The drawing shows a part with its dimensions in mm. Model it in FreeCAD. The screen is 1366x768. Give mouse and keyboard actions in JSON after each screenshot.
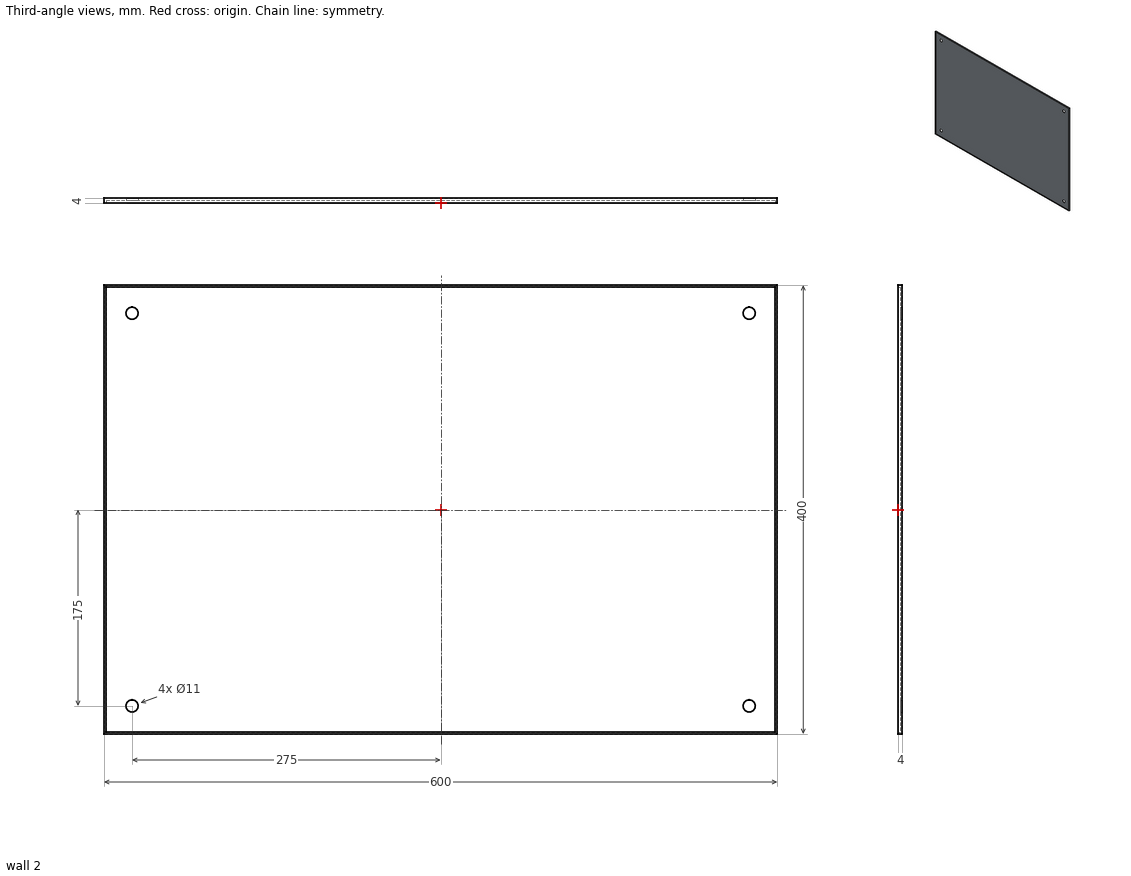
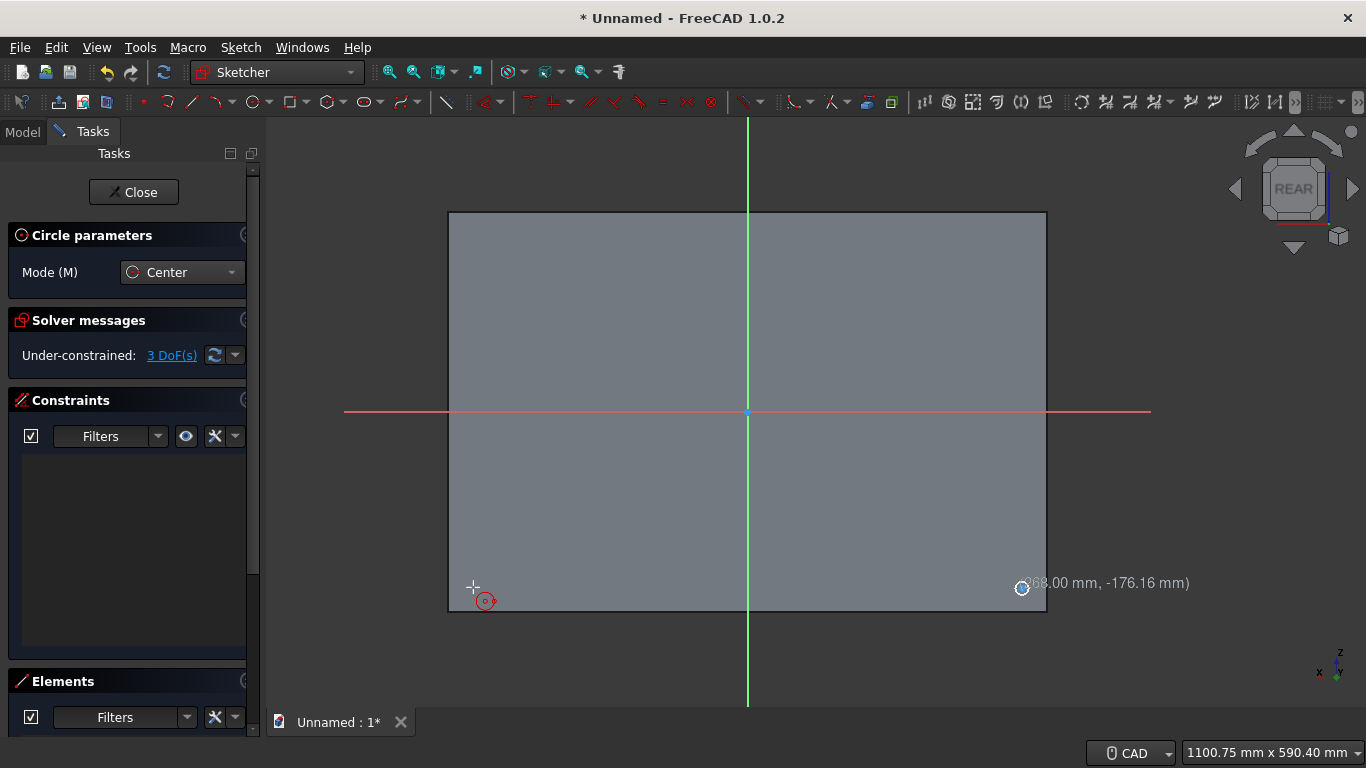
{"action": "left_click", "coordinate": [473, 587]}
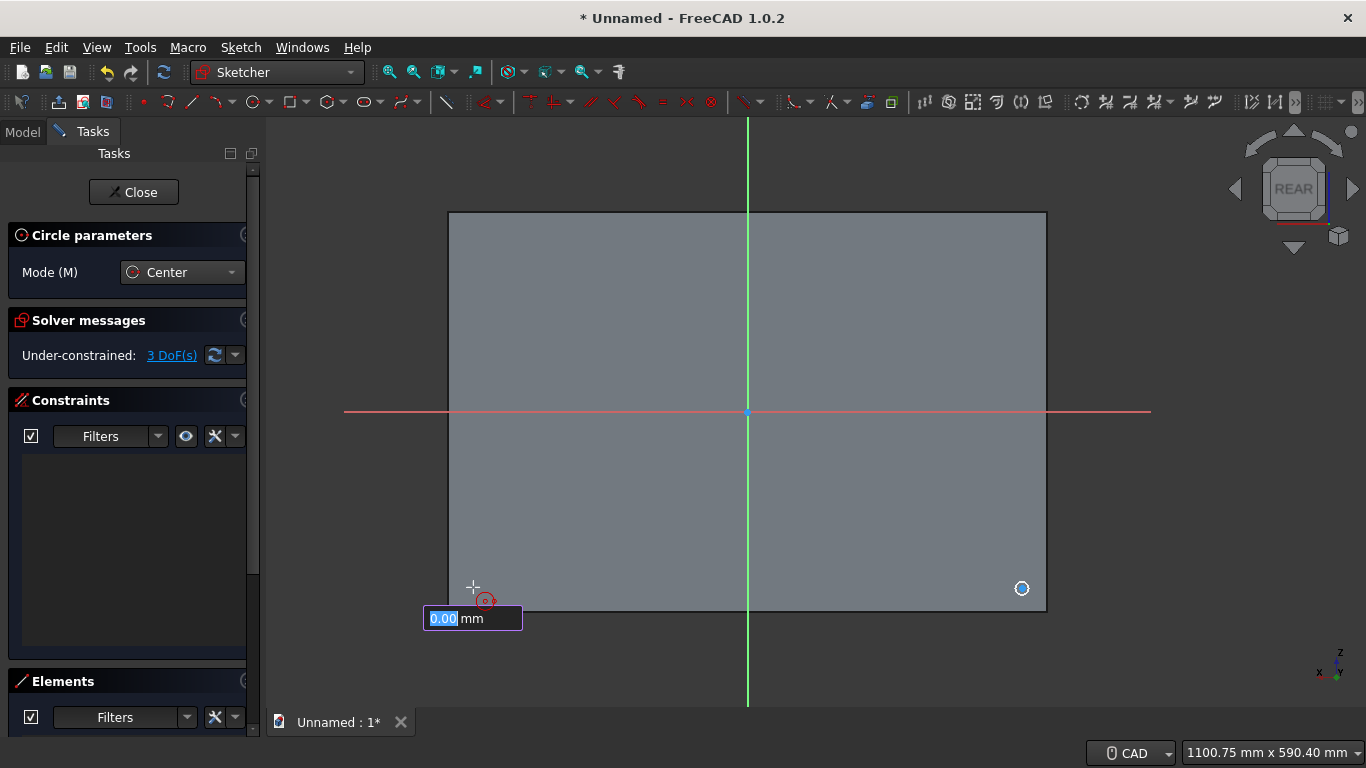
{"action": "scroll", "coordinate": [477, 583], "scroll_direction": "up", "scroll_amount": 6}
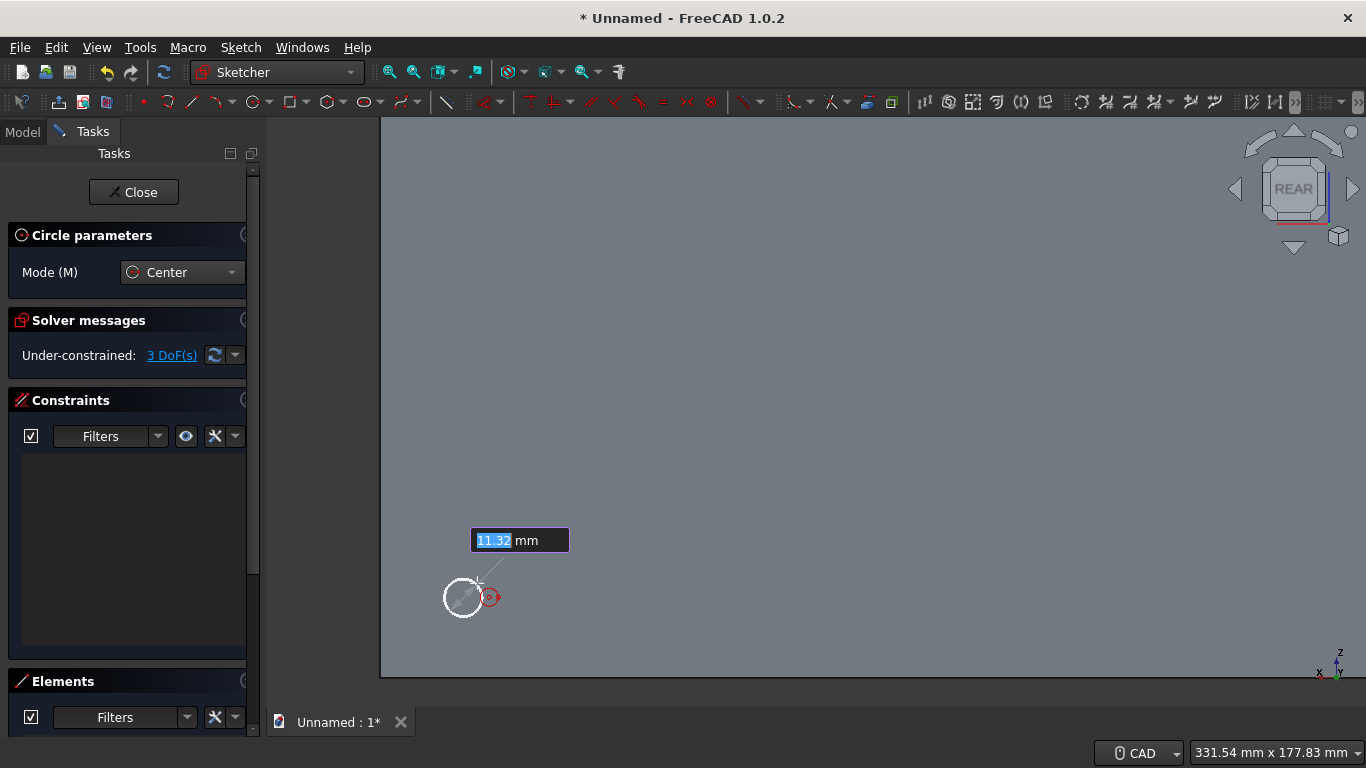
{"action": "left_click", "coordinate": [476, 582]}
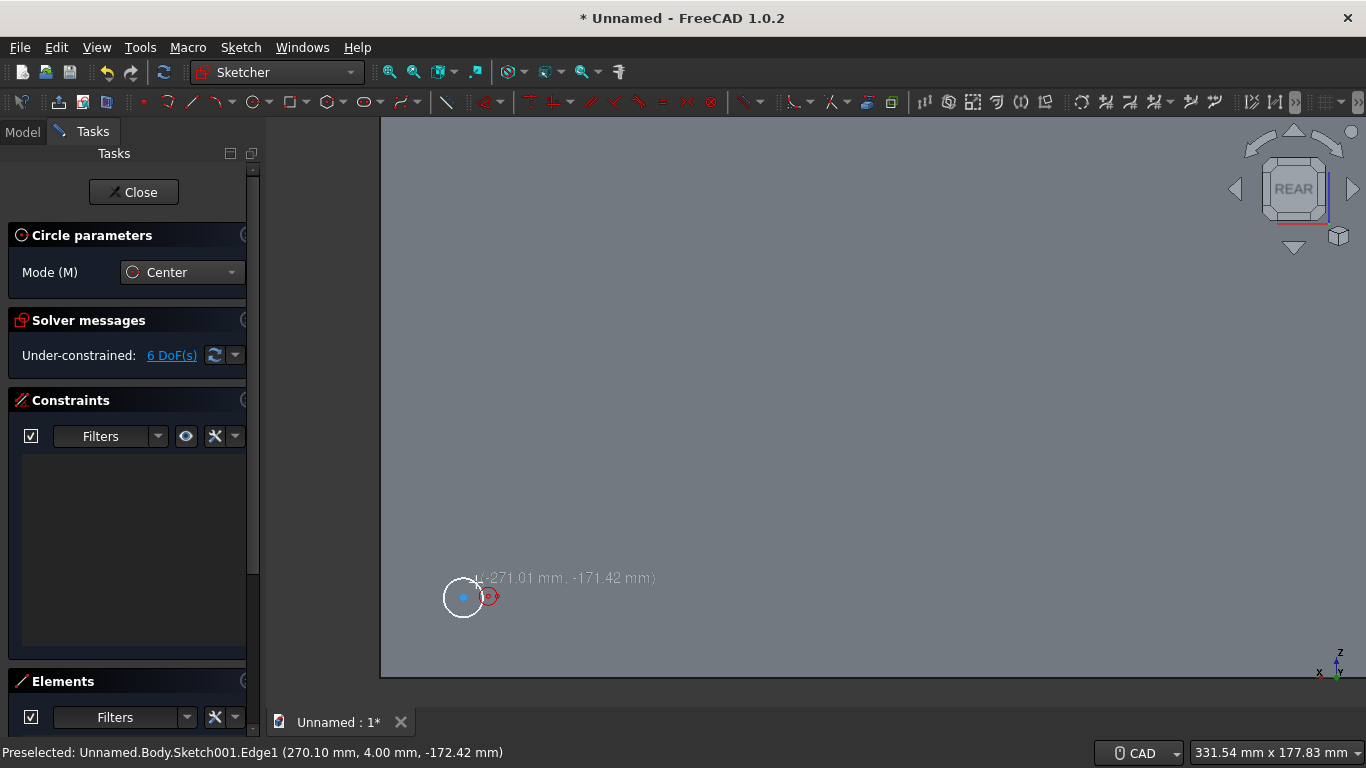
{"action": "scroll", "coordinate": [477, 583], "scroll_direction": "down", "scroll_amount": 6}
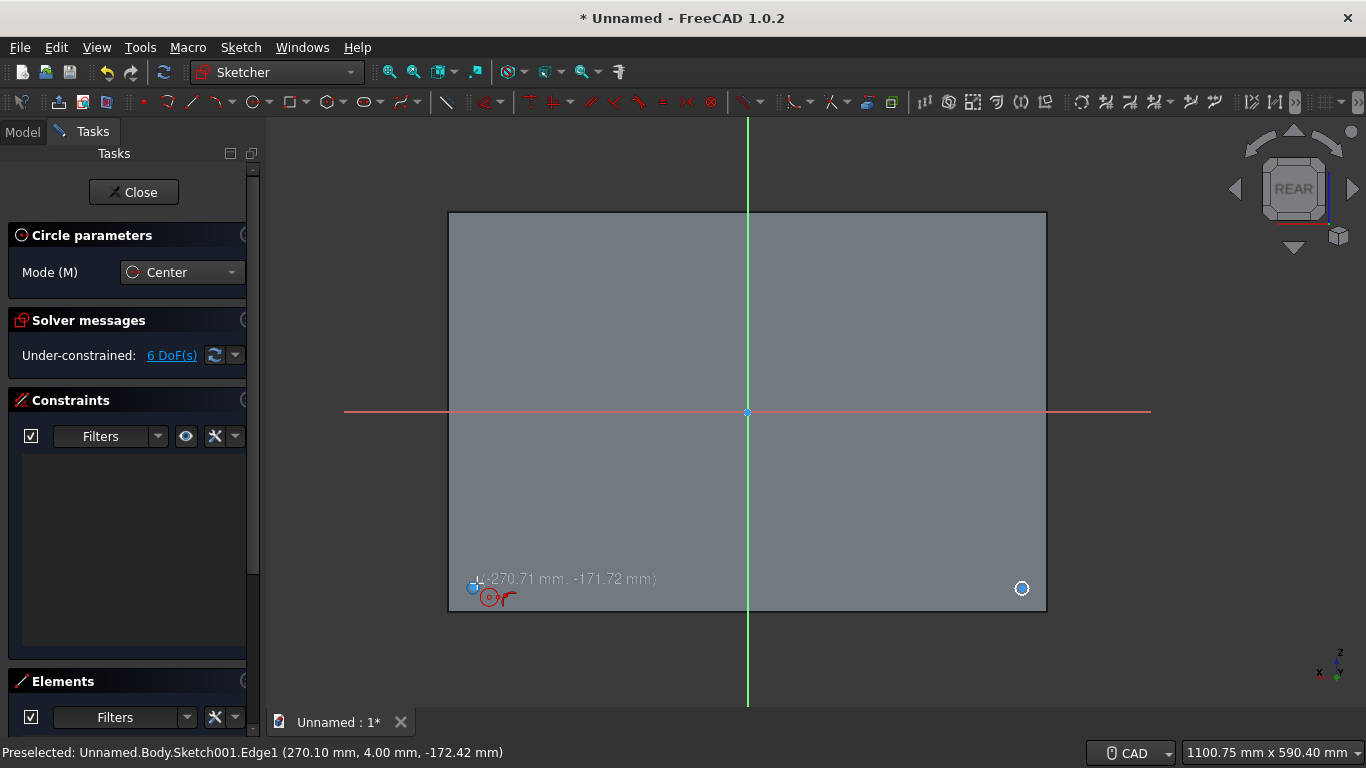
{"action": "scroll", "coordinate": [473, 237], "scroll_direction": "up", "scroll_amount": 8}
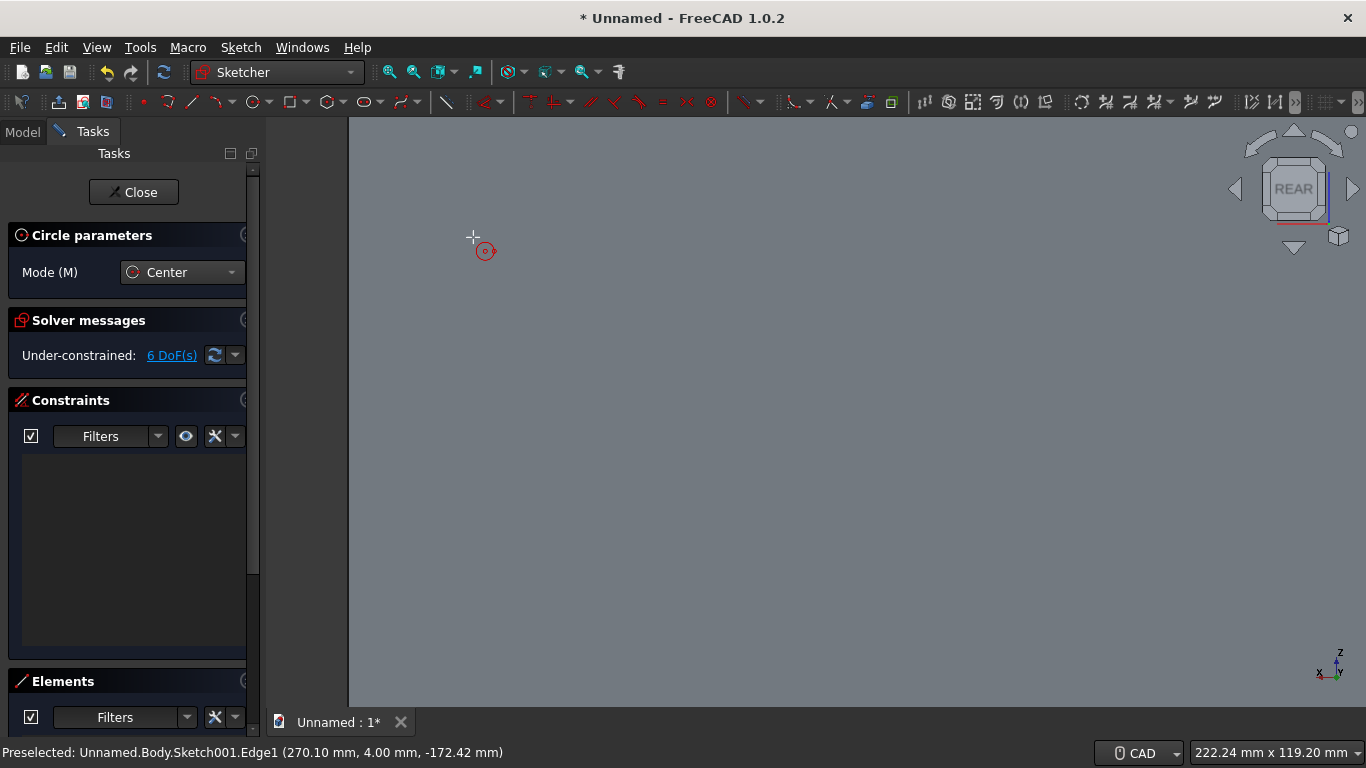
{"action": "scroll", "coordinate": [473, 237], "scroll_direction": "down", "scroll_amount": 8}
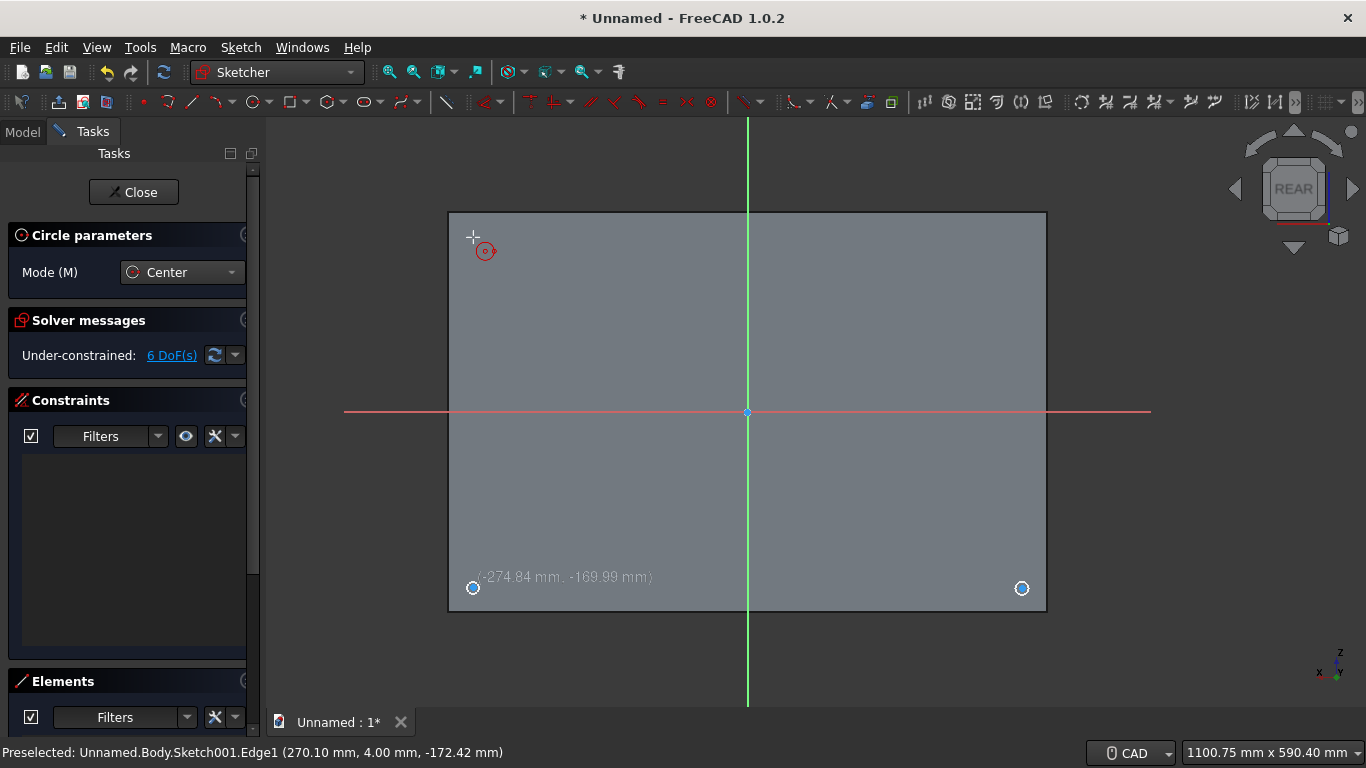
{"action": "left_click", "coordinate": [473, 237]}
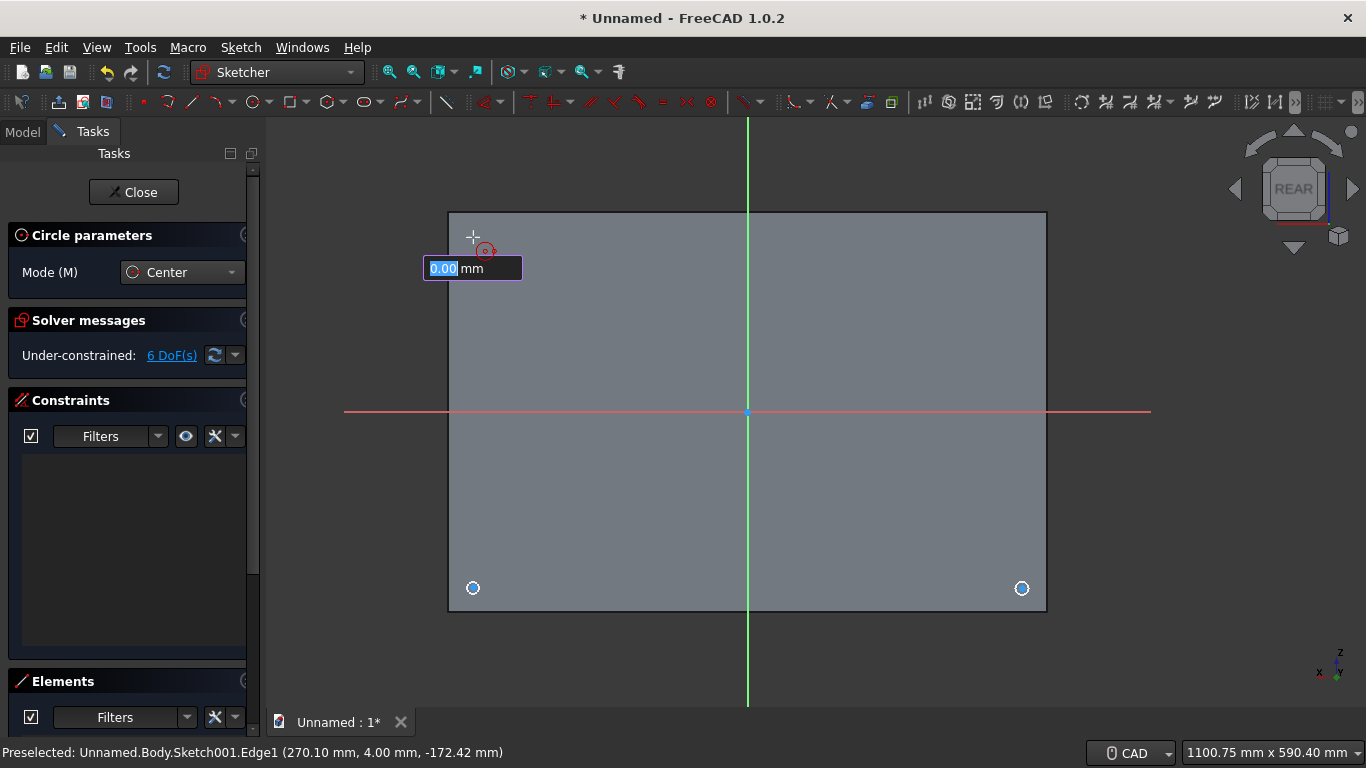
{"action": "scroll", "coordinate": [477, 233], "scroll_direction": "up", "scroll_amount": 6}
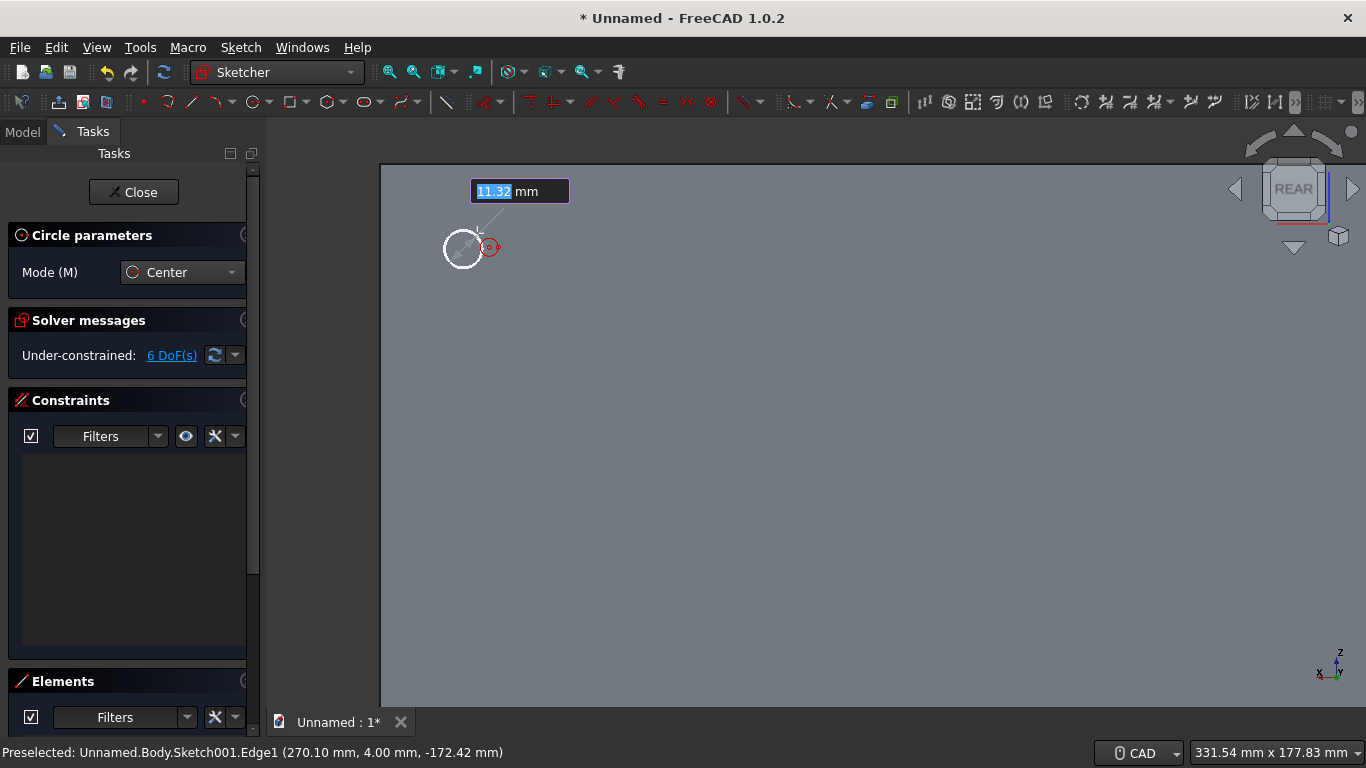
{"action": "left_click", "coordinate": [476, 234]}